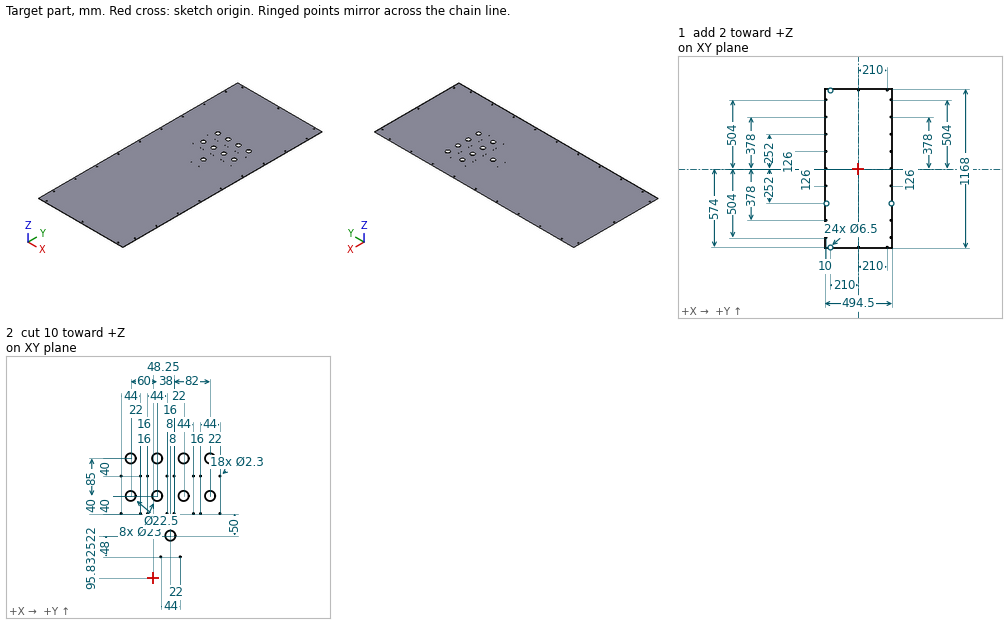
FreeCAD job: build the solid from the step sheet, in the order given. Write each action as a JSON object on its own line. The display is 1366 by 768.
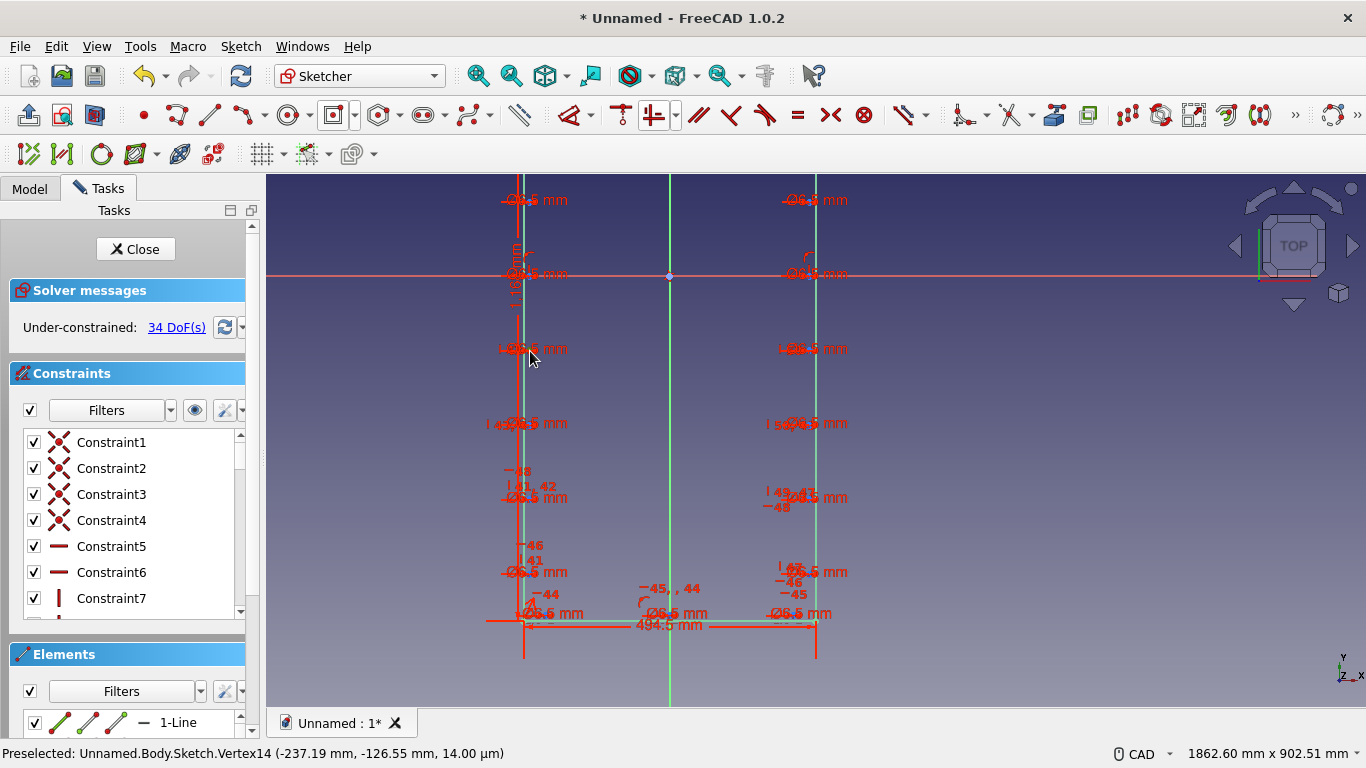
{"action": "left_click", "coordinate": [530, 276]}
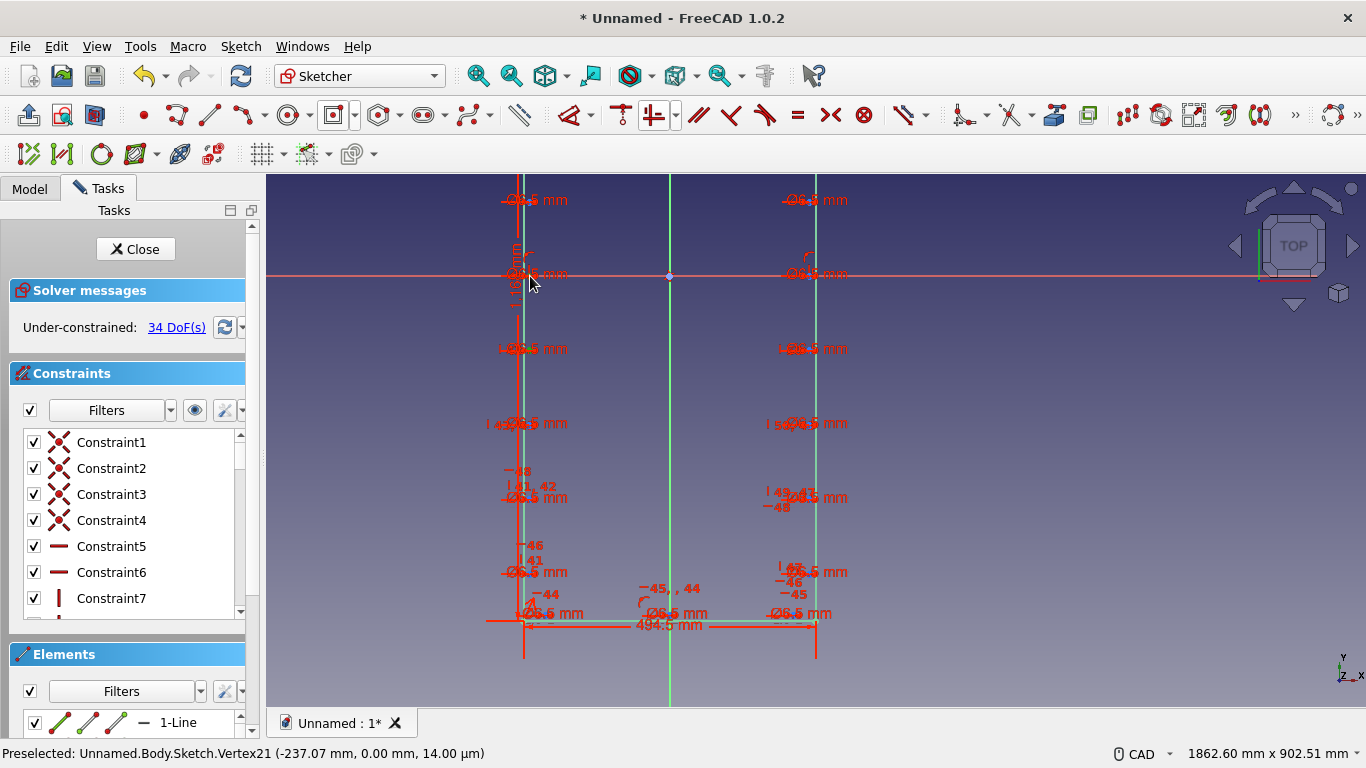
{"action": "left_click", "coordinate": [676, 116]}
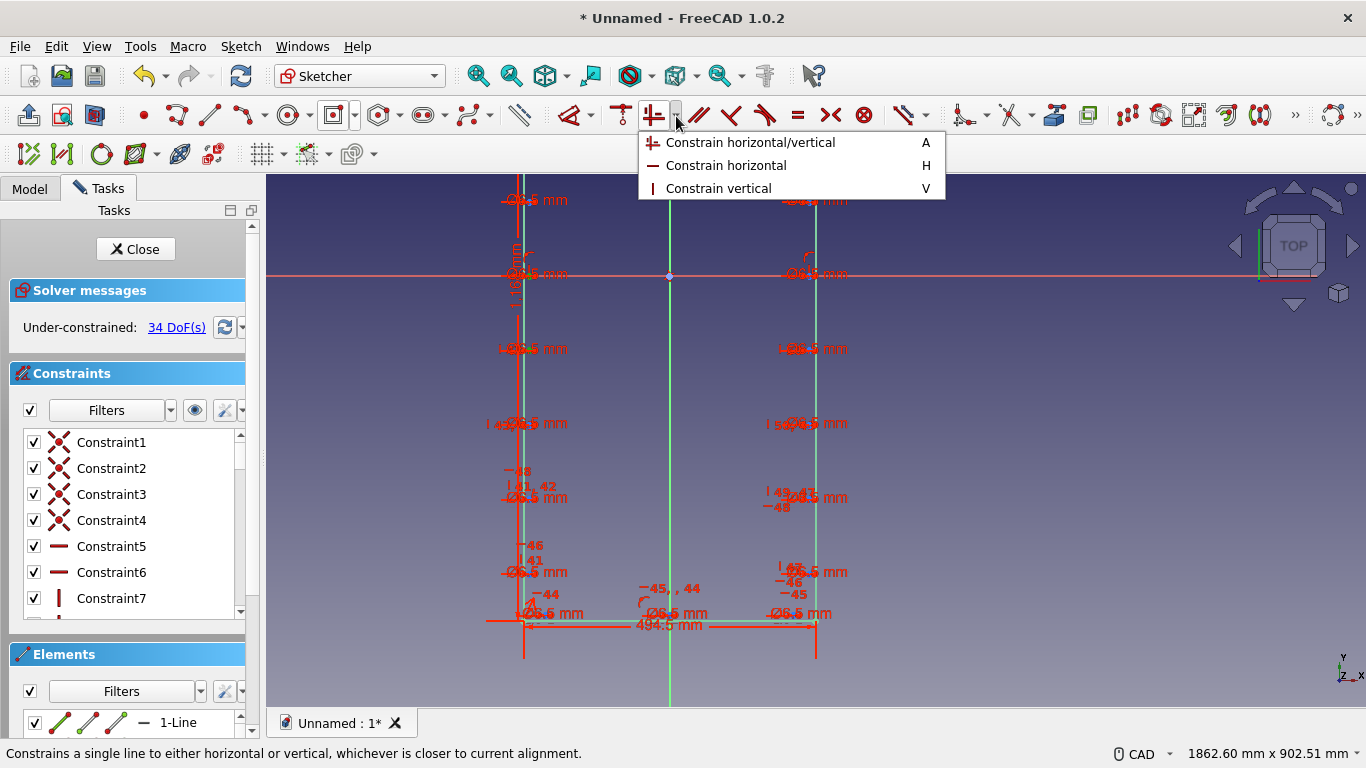
{"action": "left_click", "coordinate": [792, 188]}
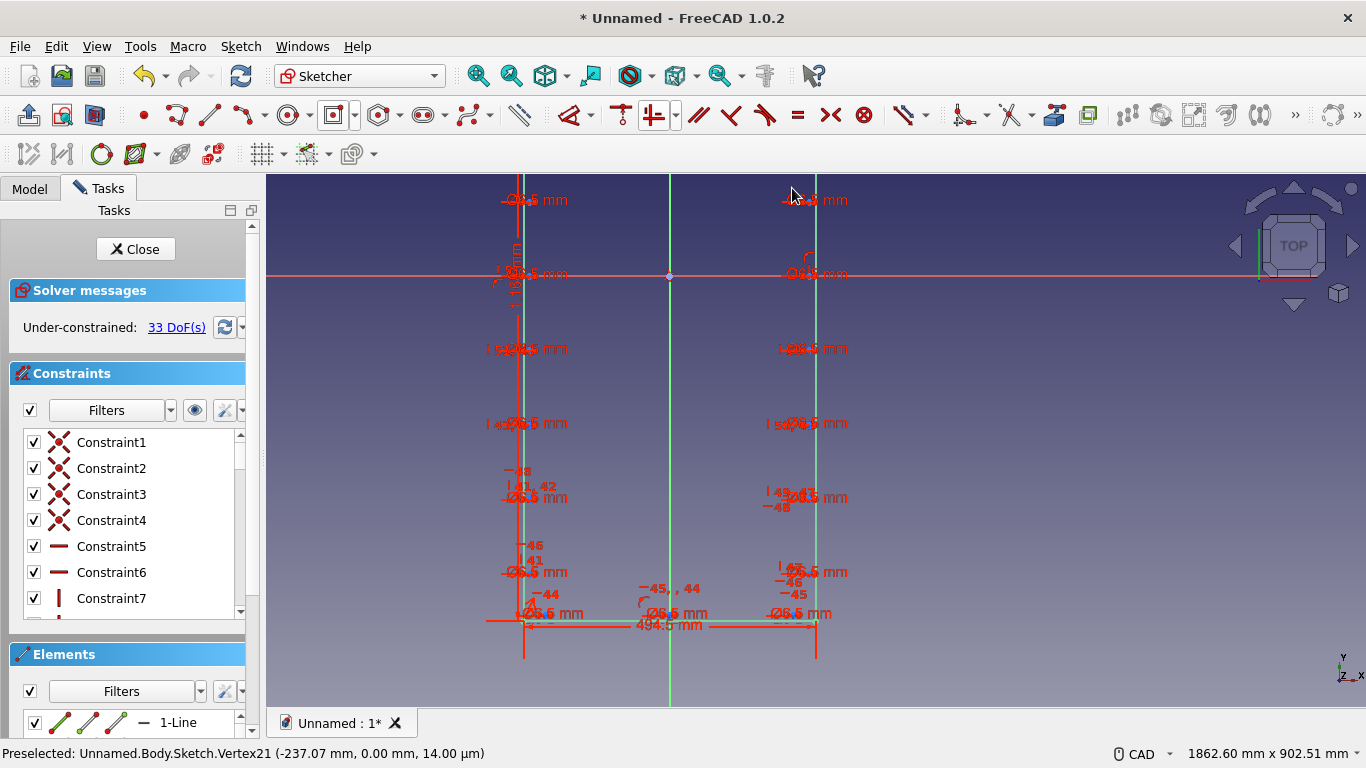
{"action": "left_click", "coordinate": [530, 276]}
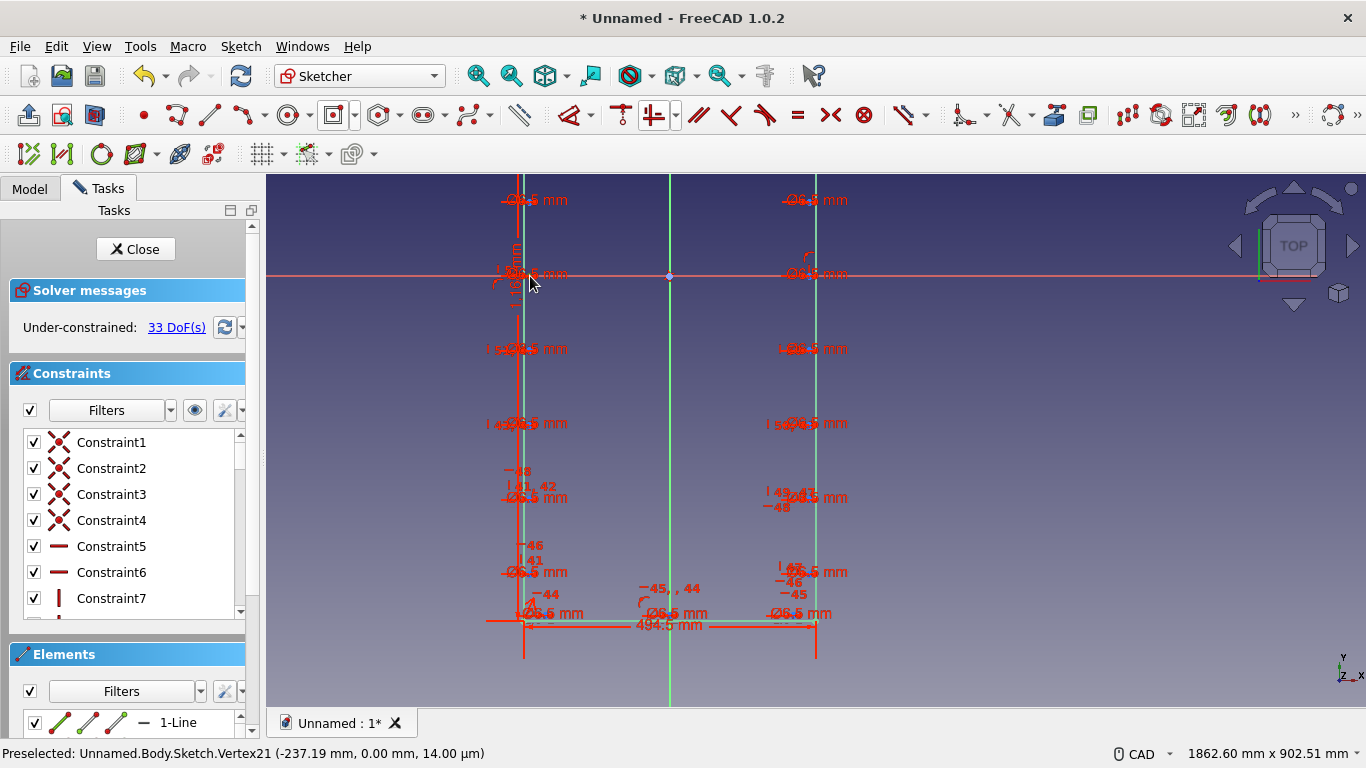
{"action": "left_click", "coordinate": [530, 202]}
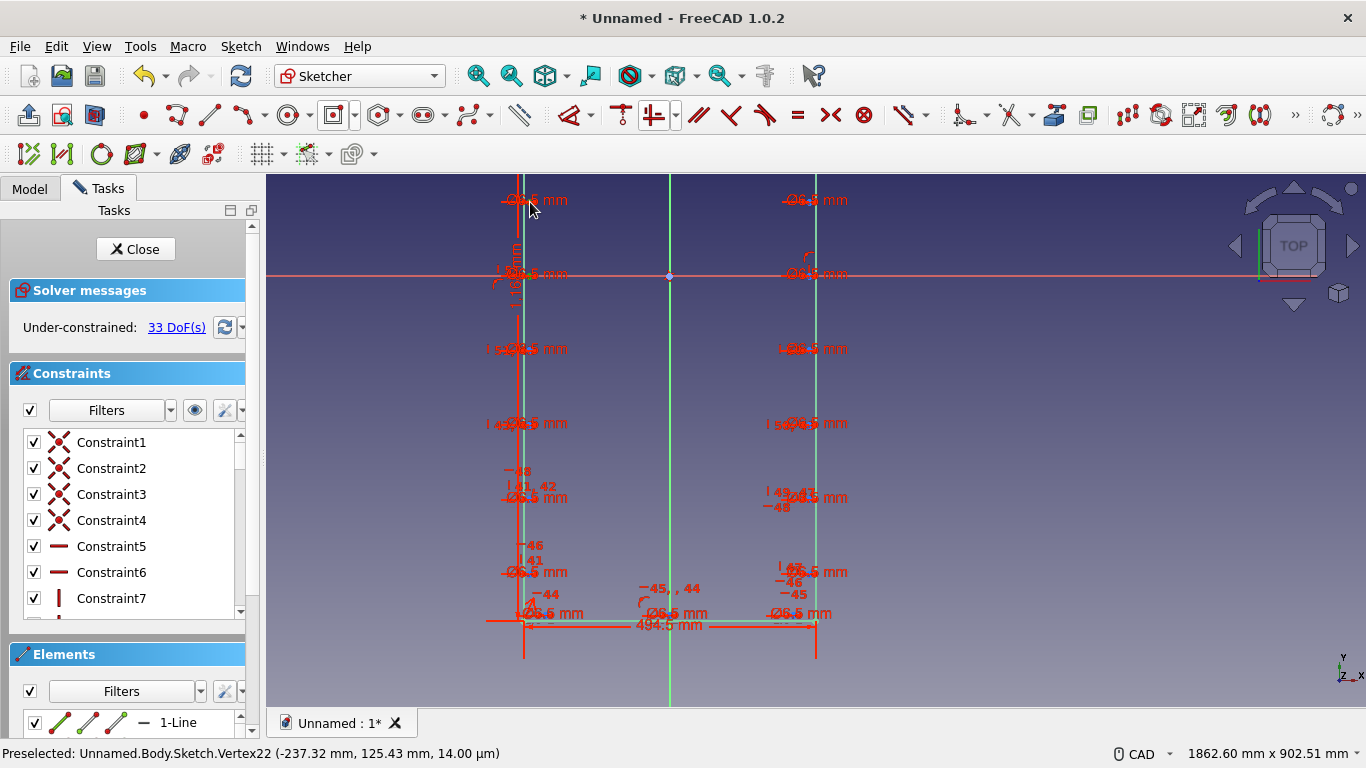
{"action": "key", "text": "v"}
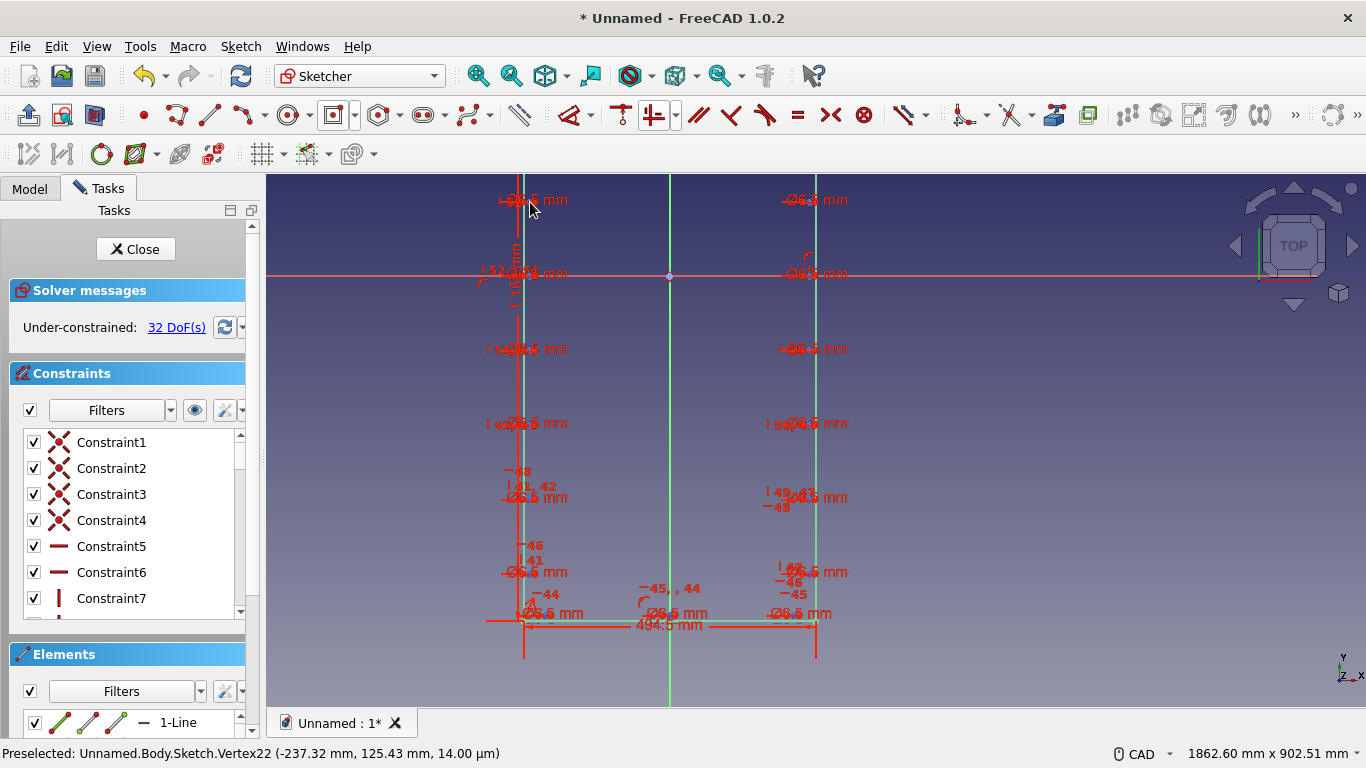
{"action": "left_click", "coordinate": [530, 202]}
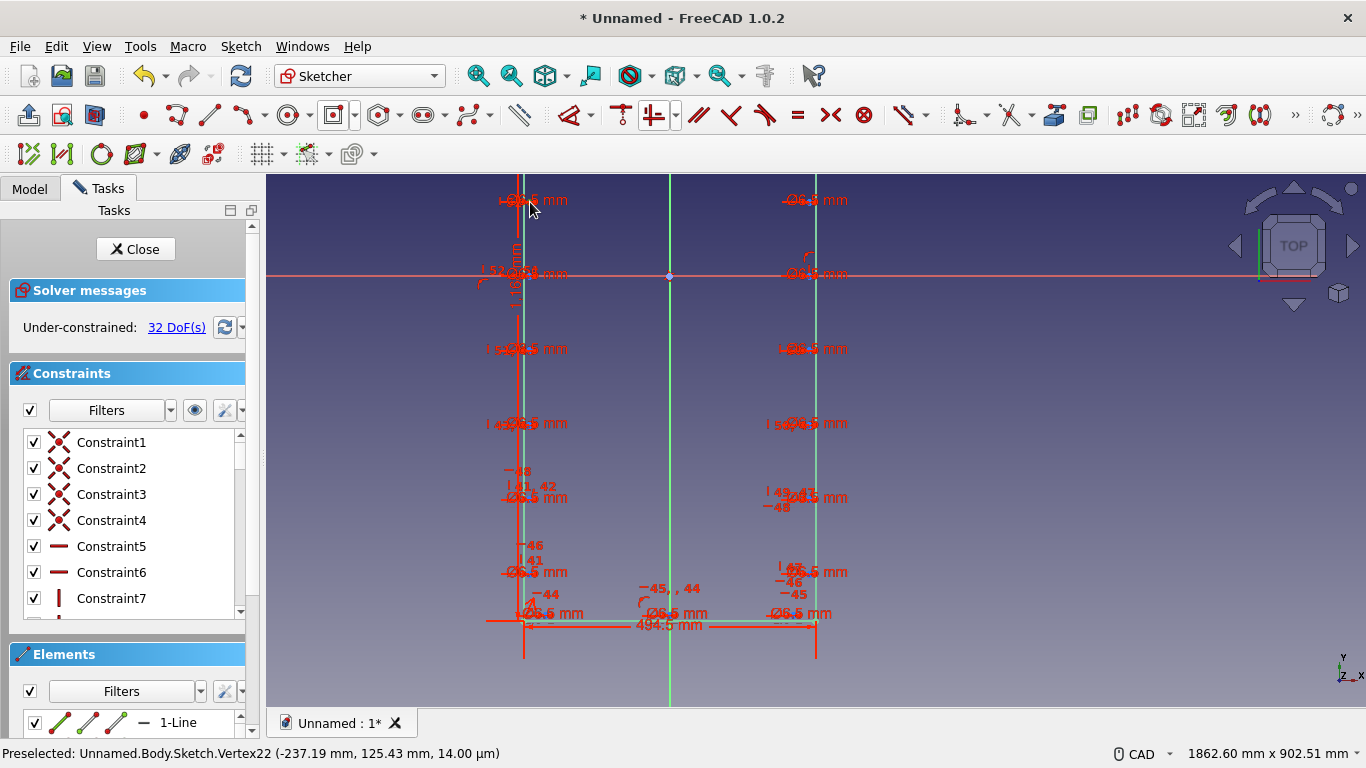
{"action": "scroll", "coordinate": [811, 575], "scroll_direction": "down", "scroll_amount": 4}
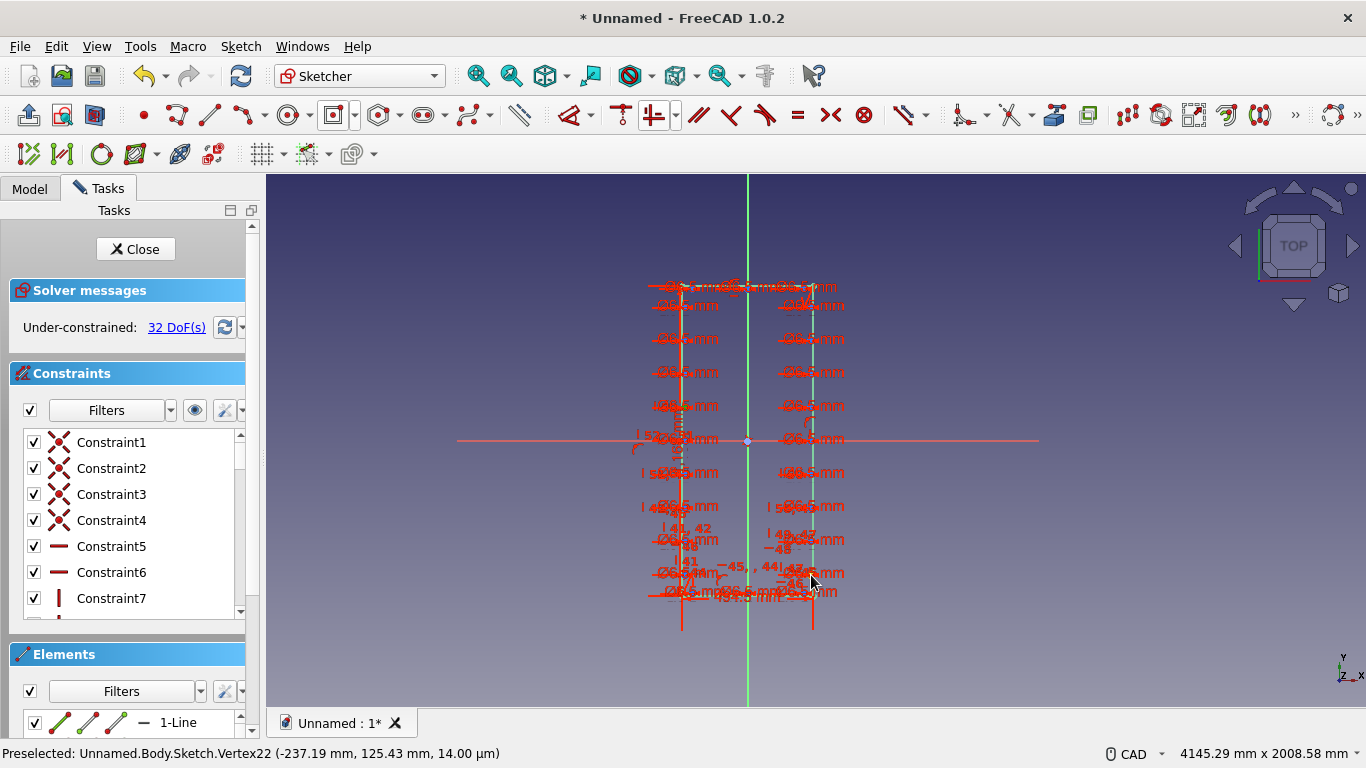
{"action": "left_click", "coordinate": [685, 374]}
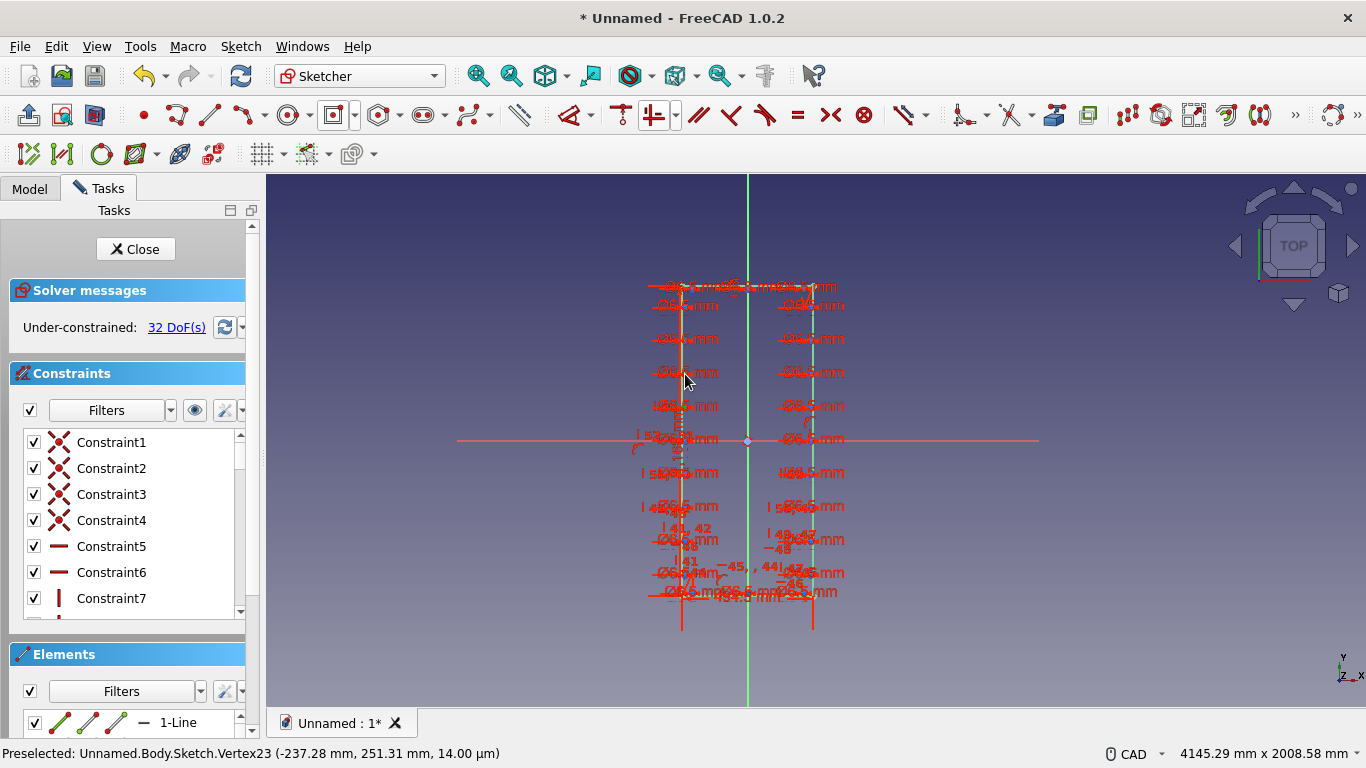
{"action": "left_click", "coordinate": [676, 116]}